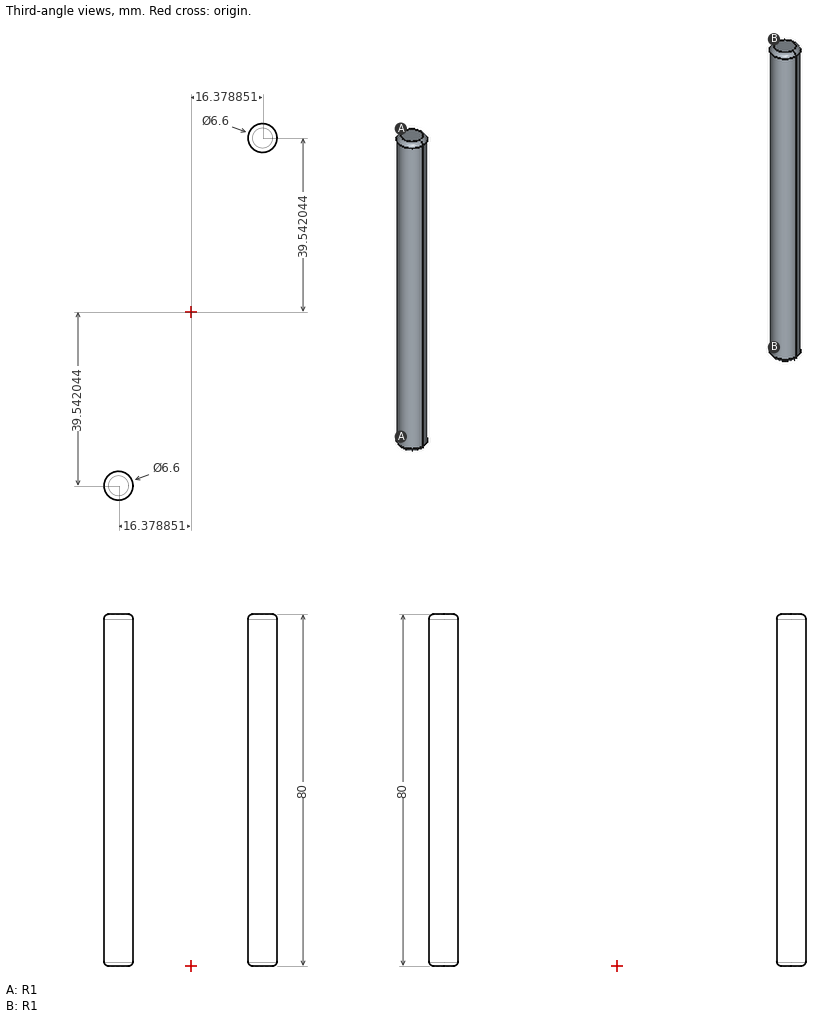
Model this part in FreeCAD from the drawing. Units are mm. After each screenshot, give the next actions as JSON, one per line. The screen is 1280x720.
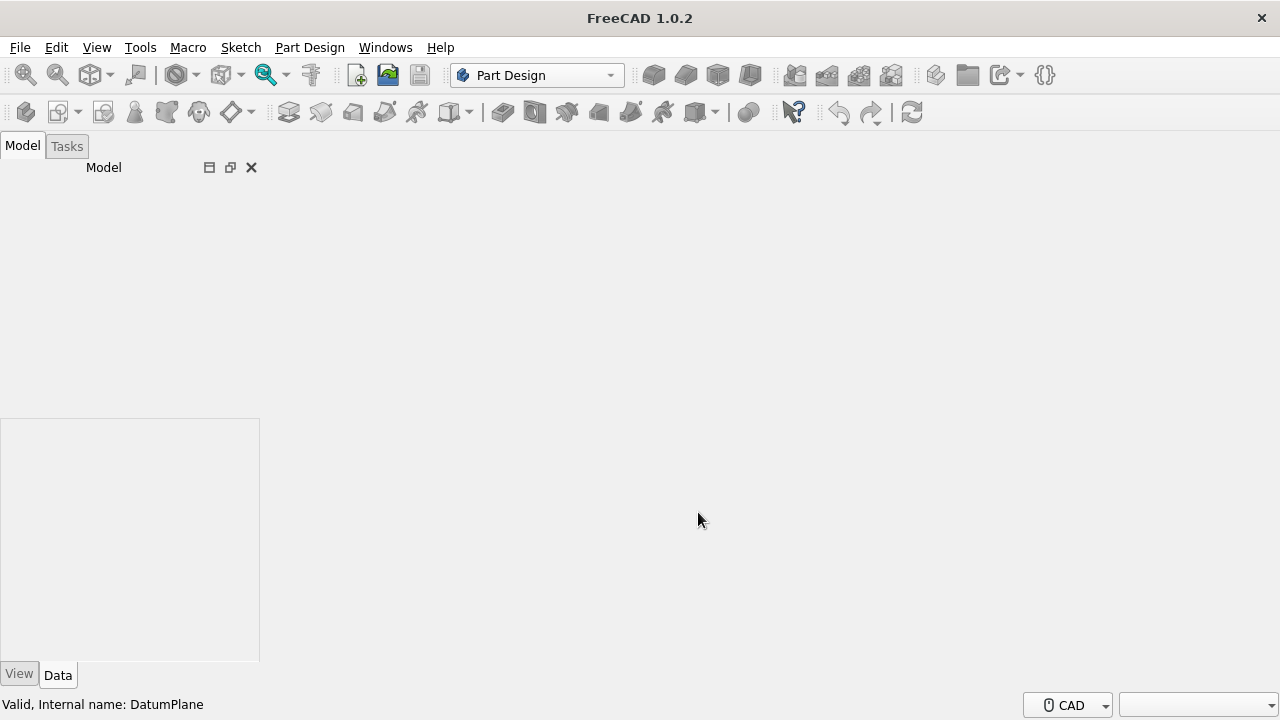
{"action": "key", "text": "ctrl+n"}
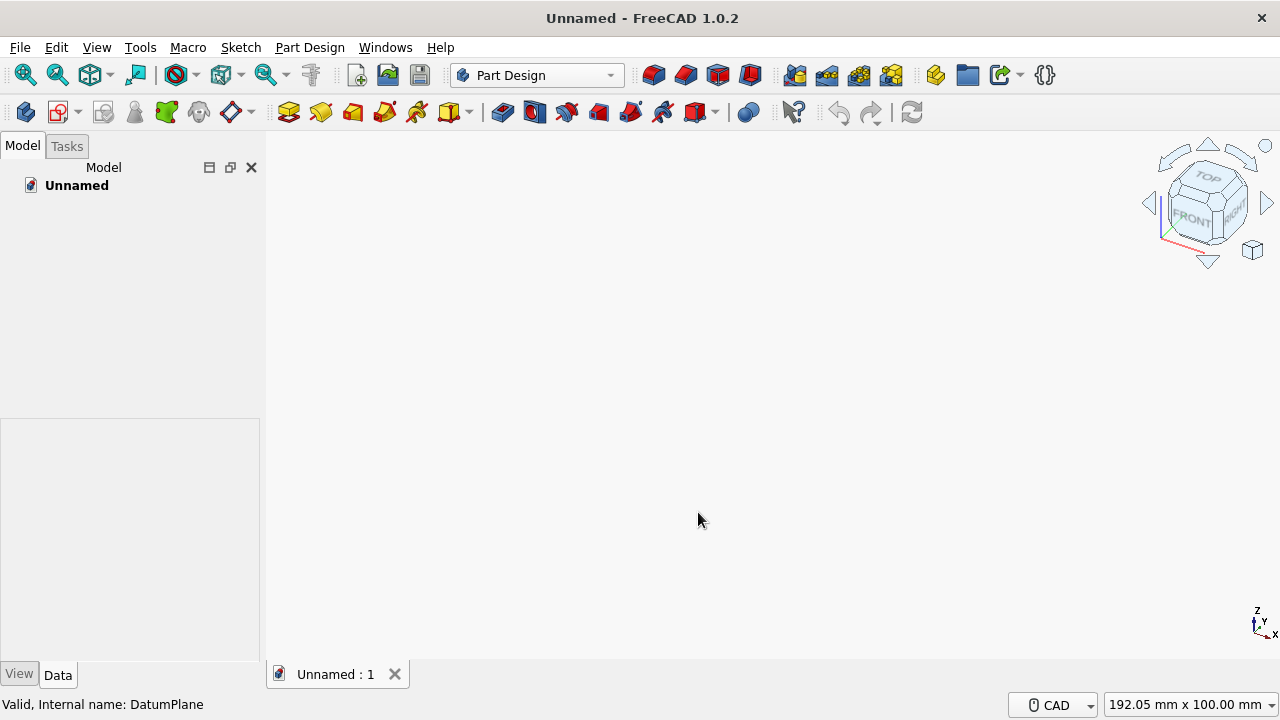
{"action": "left_click", "coordinate": [58, 112]}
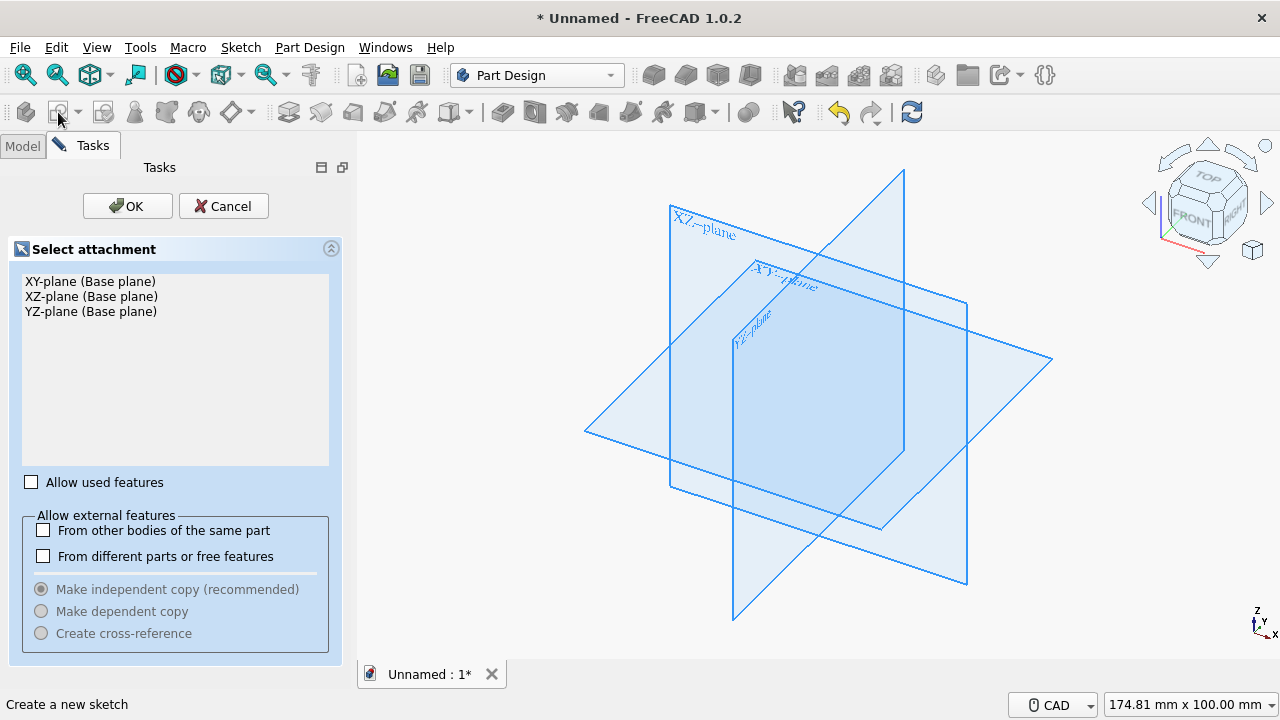
{"action": "left_click", "coordinate": [82, 282]}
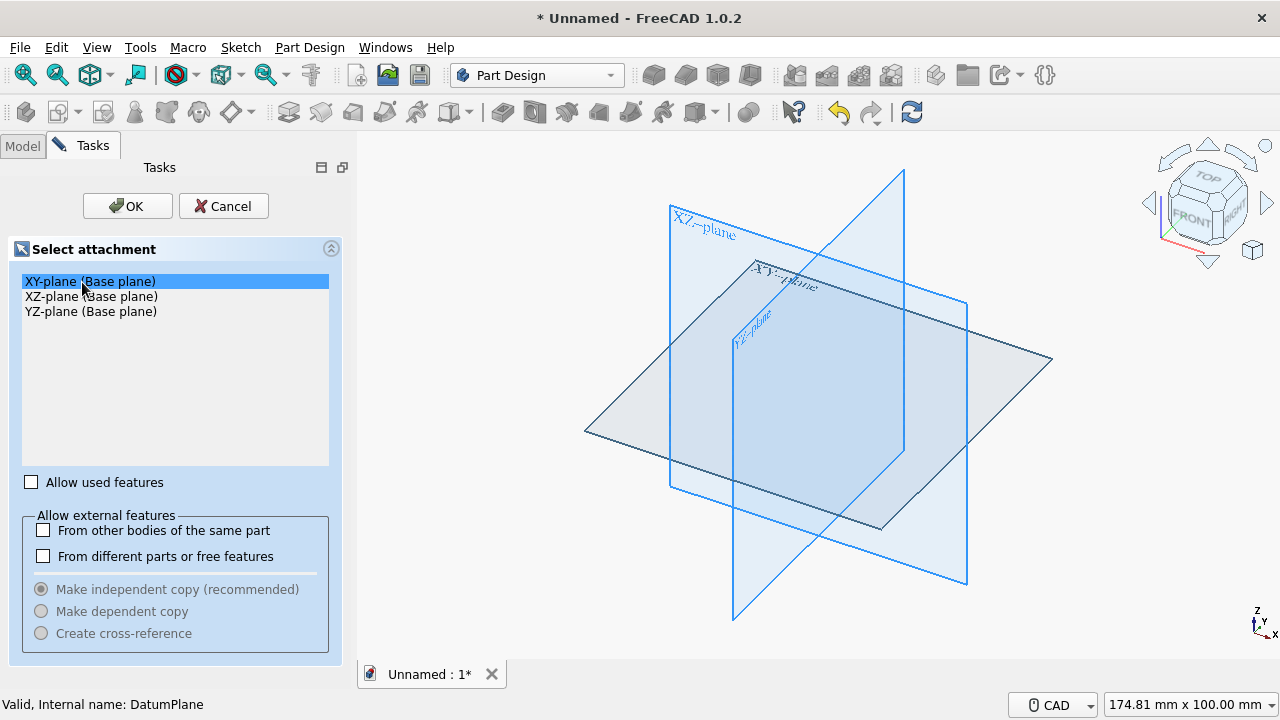
{"action": "left_click", "coordinate": [128, 206]}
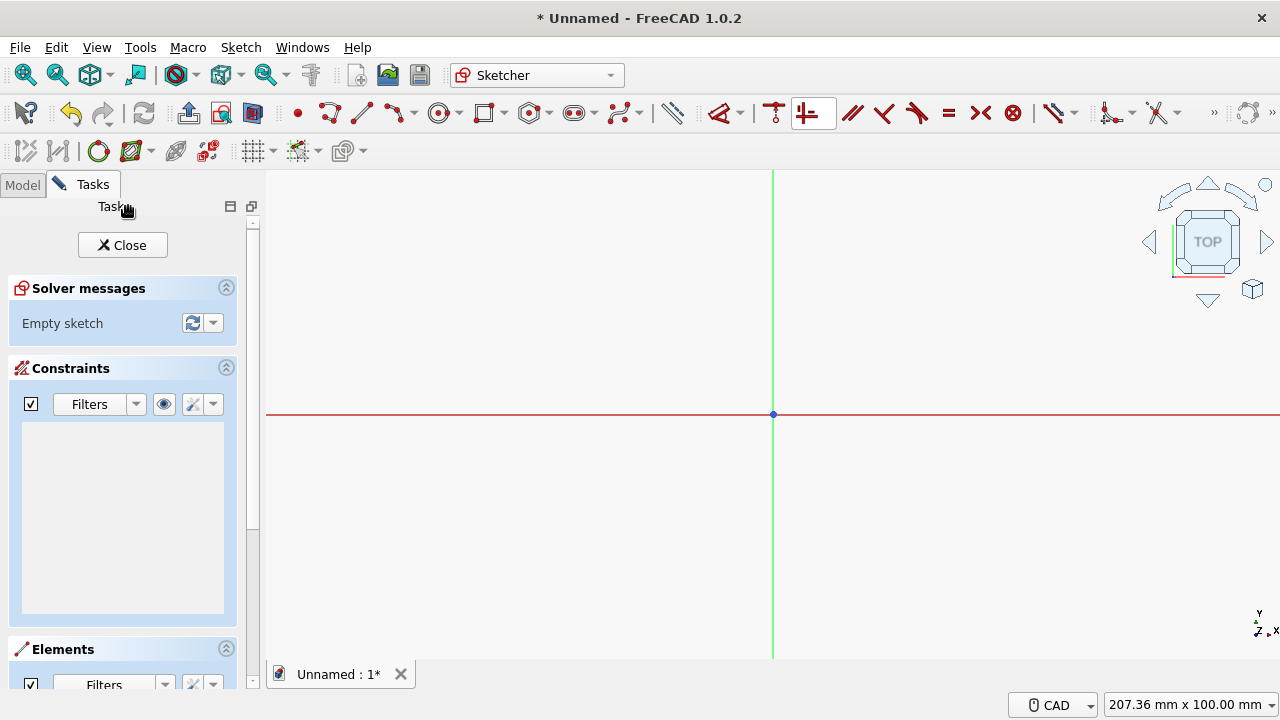
{"action": "scroll", "coordinate": [691, 631], "scroll_direction": "up", "scroll_amount": 11}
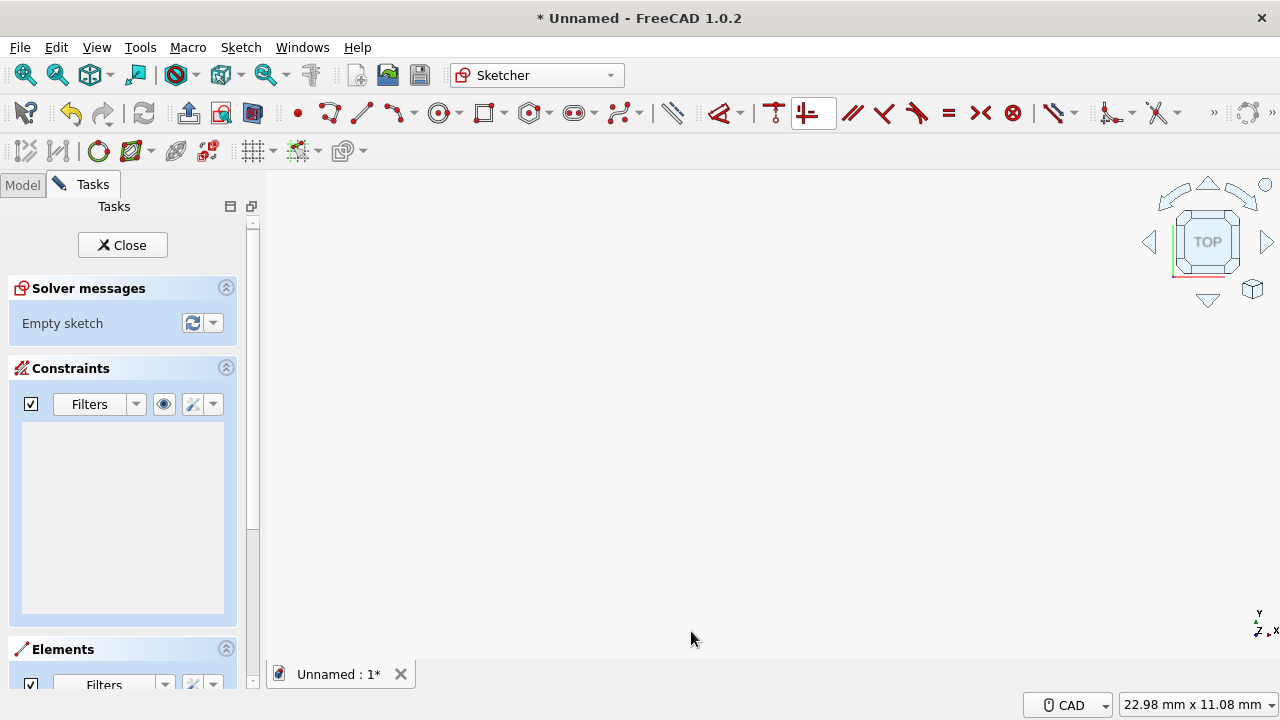
{"action": "left_click", "coordinate": [440, 114]}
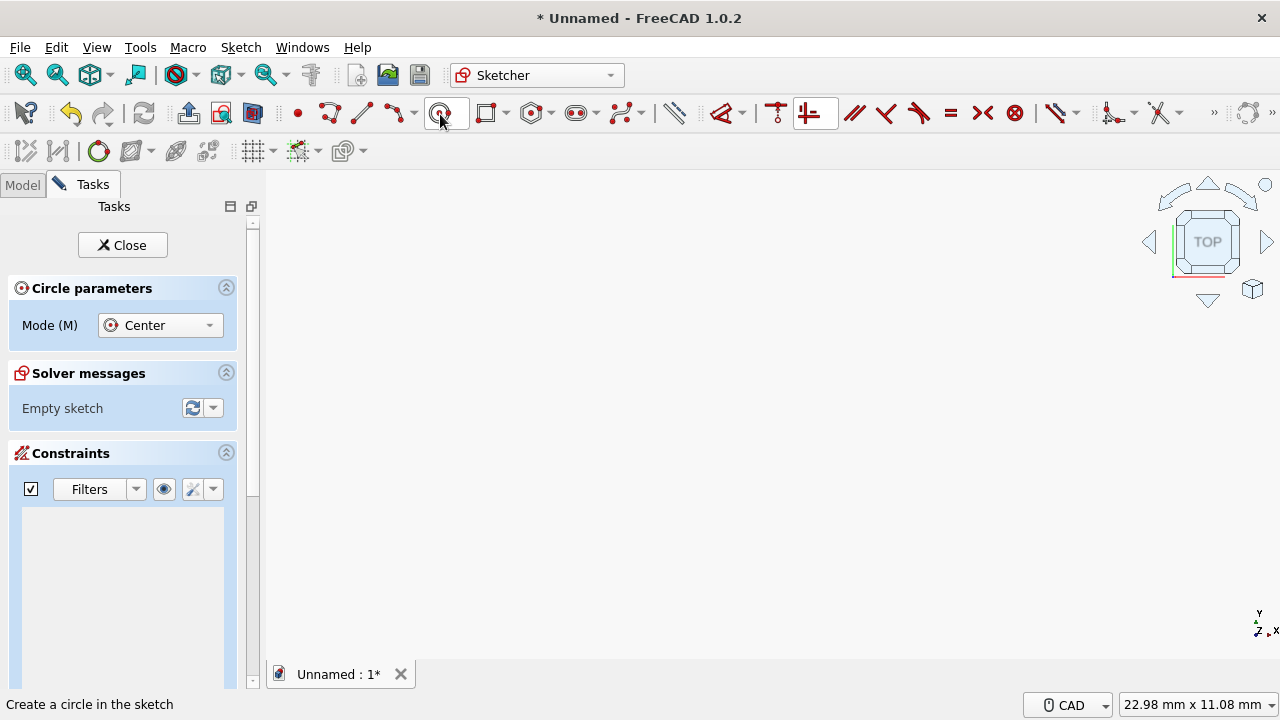
{"action": "left_click", "coordinate": [705, 415]}
{"action": "left_click", "coordinate": [808, 312]}
{"action": "key", "text": "Escape"}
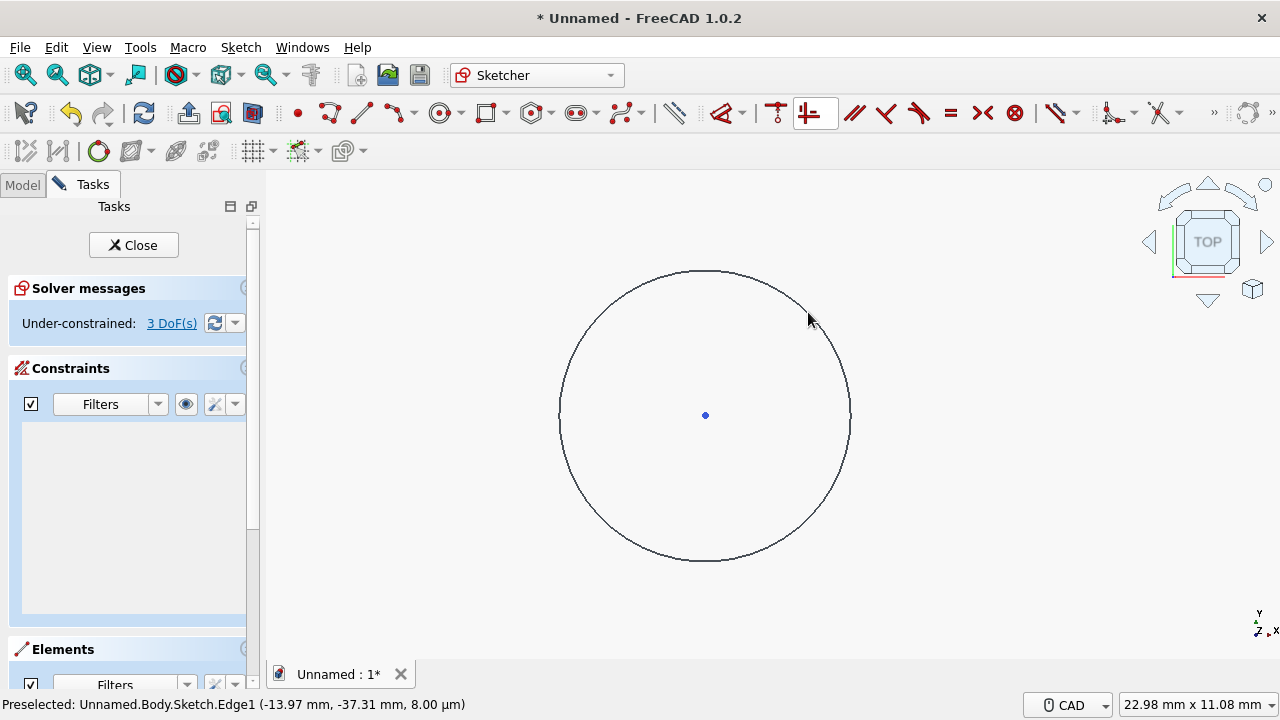
{"action": "left_click", "coordinate": [722, 114]}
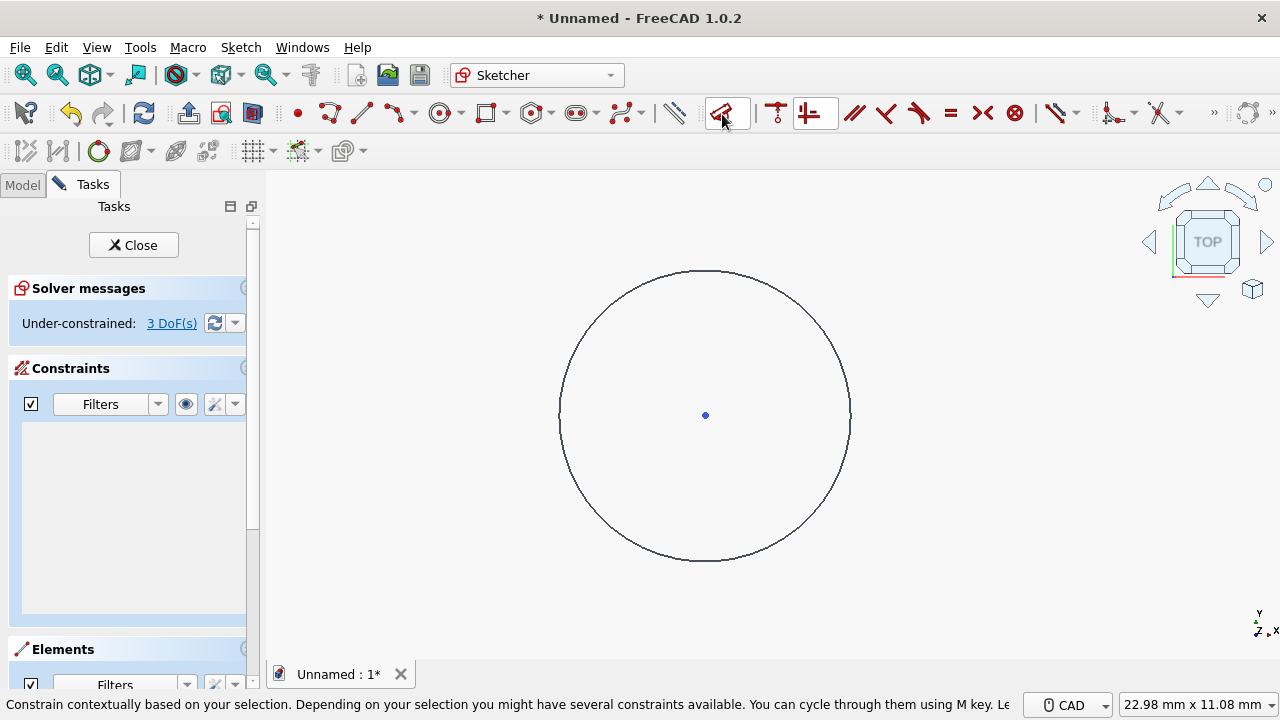
{"action": "left_click", "coordinate": [808, 313]}
{"action": "left_click", "coordinate": [831, 290]}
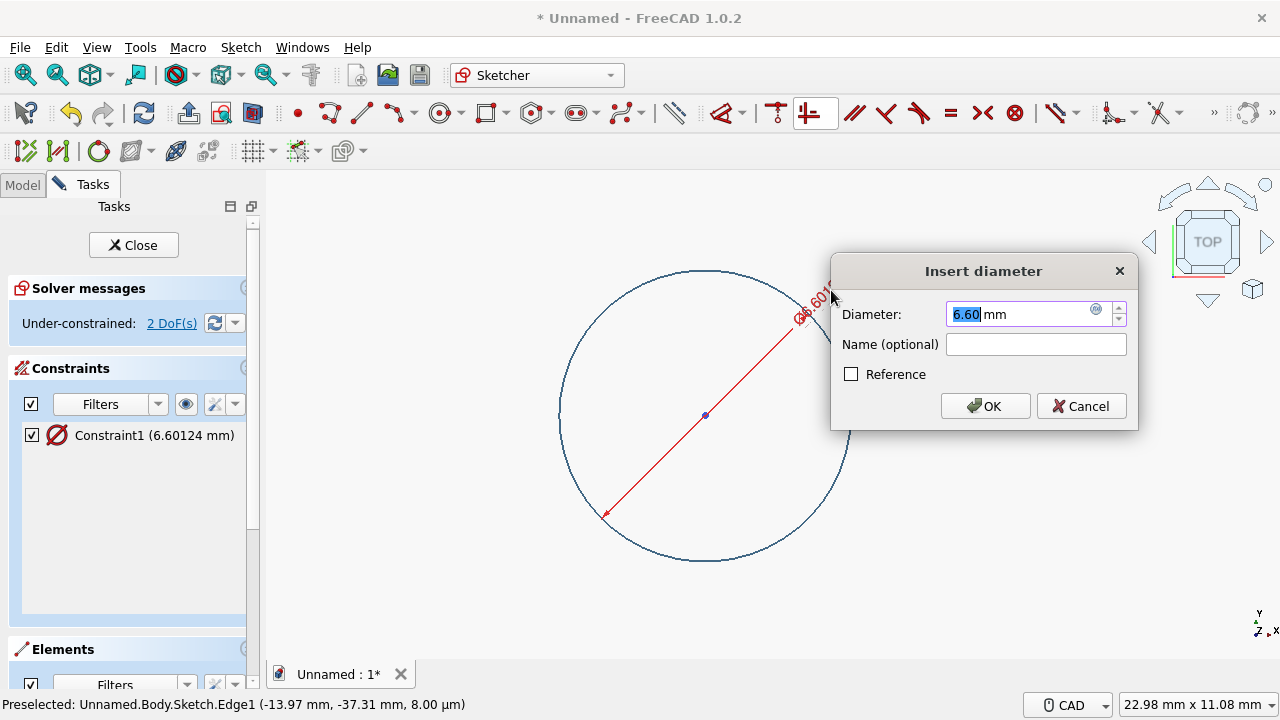
{"action": "type", "text": "6.6"}
{"action": "key", "text": "Return"}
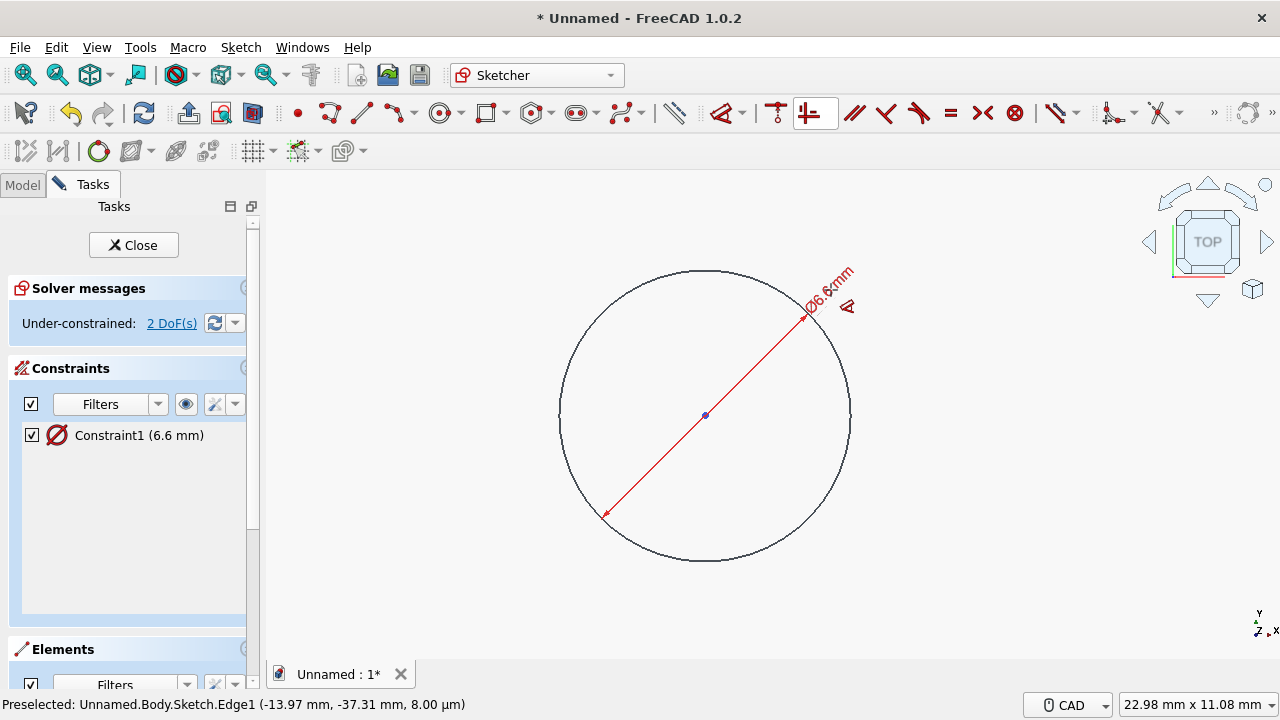
{"action": "left_click", "coordinate": [705, 416]}
{"action": "left_click", "coordinate": [910, 450]}